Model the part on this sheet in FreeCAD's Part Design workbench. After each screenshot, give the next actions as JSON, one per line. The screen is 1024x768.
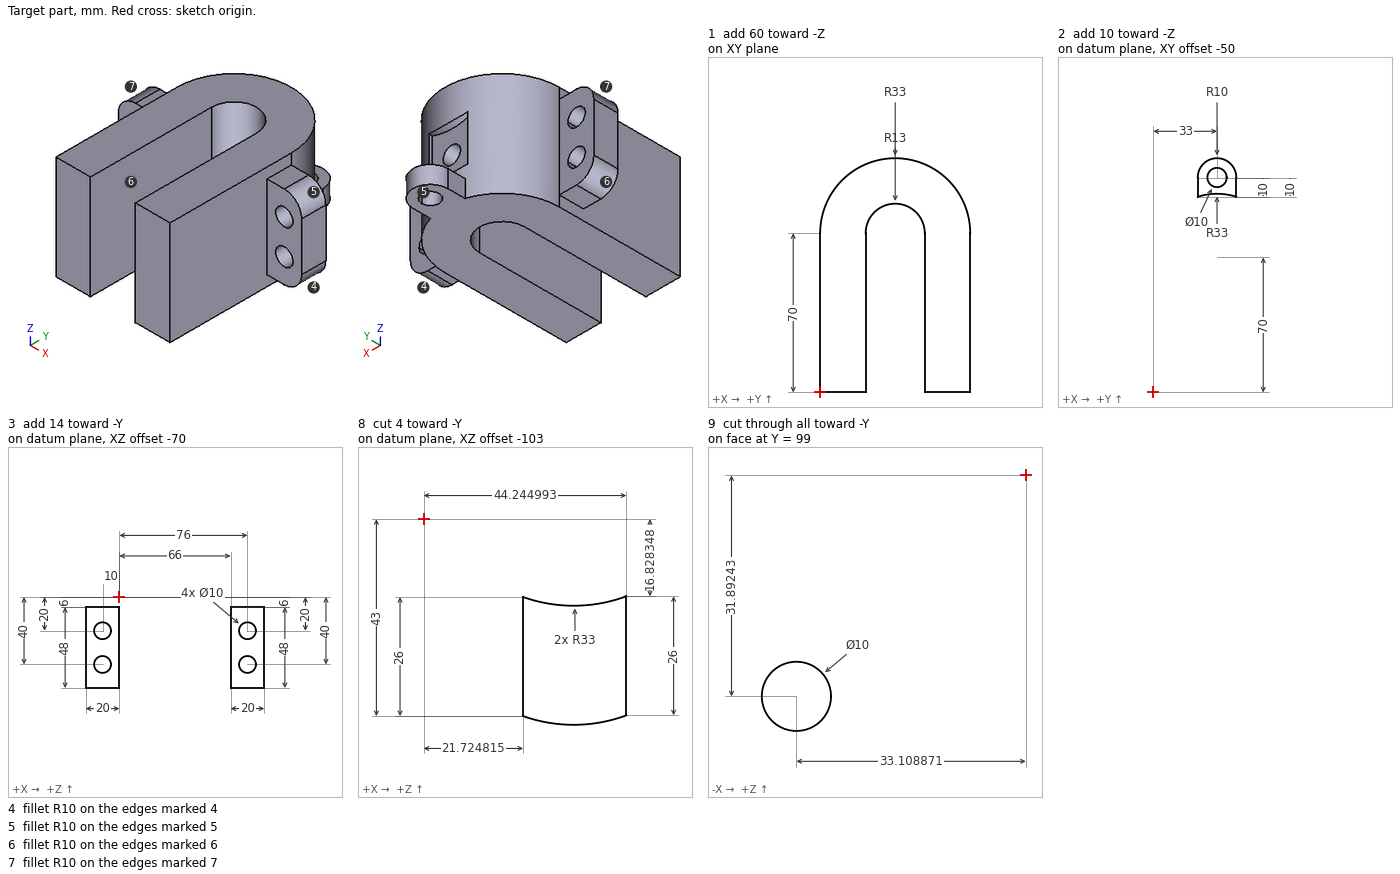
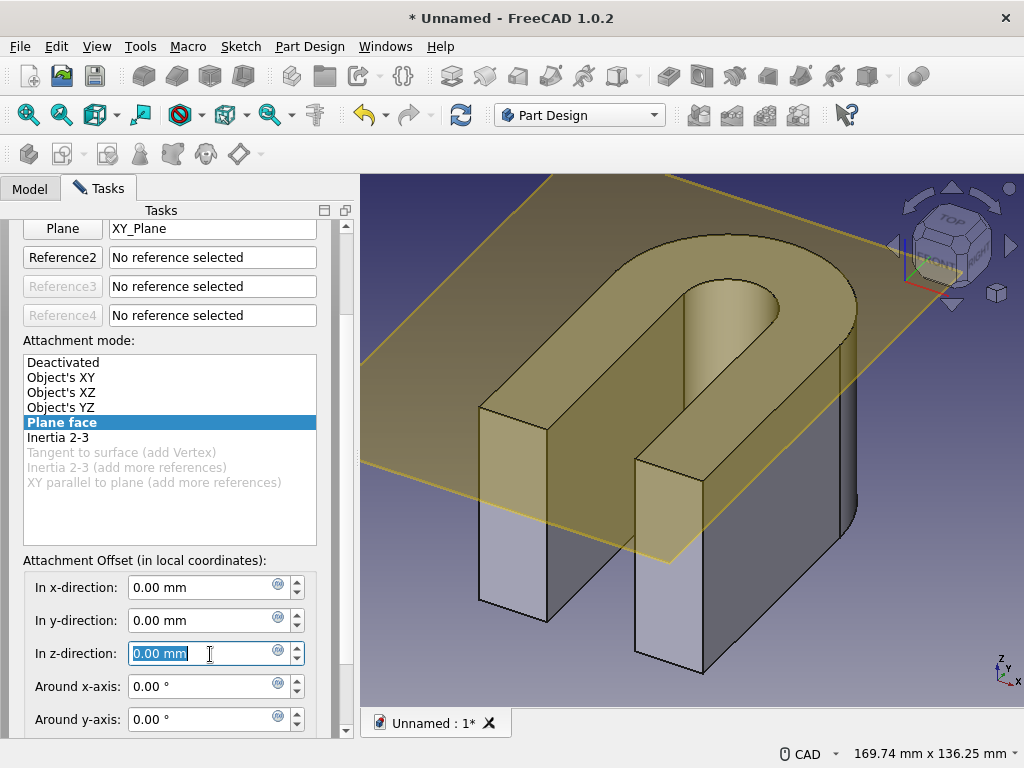
{"action": "type", "text": "-50"}
{"action": "key", "text": "Tab"}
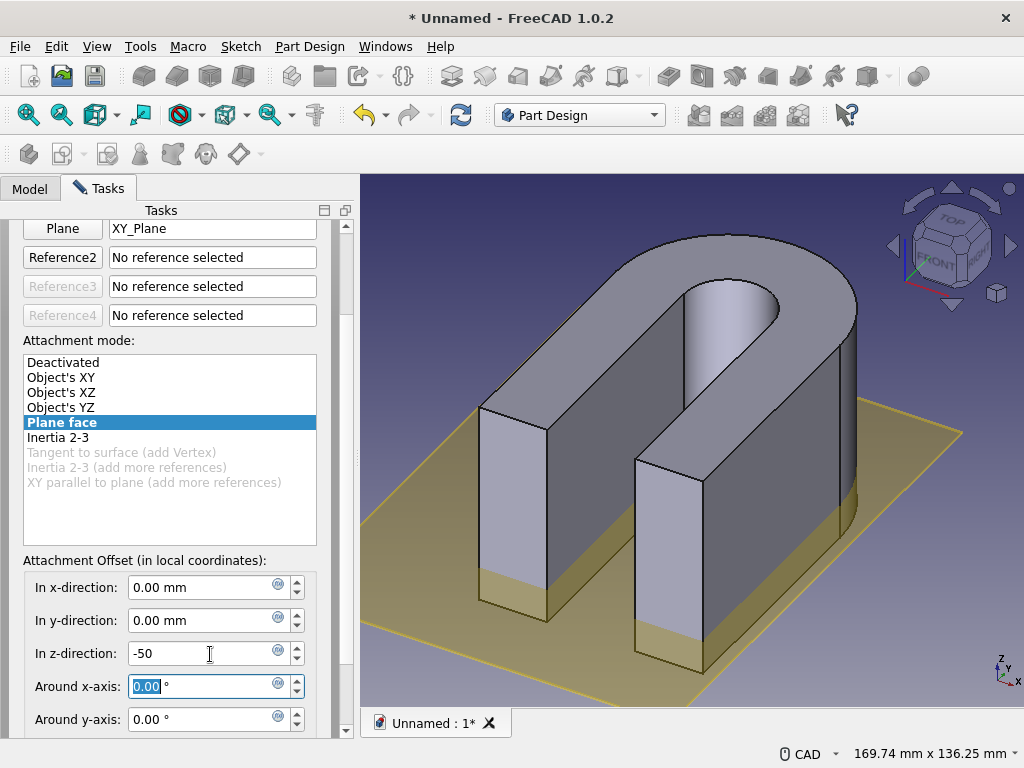
{"action": "scroll", "coordinate": [346, 479], "scroll_direction": "up", "scroll_amount": 3}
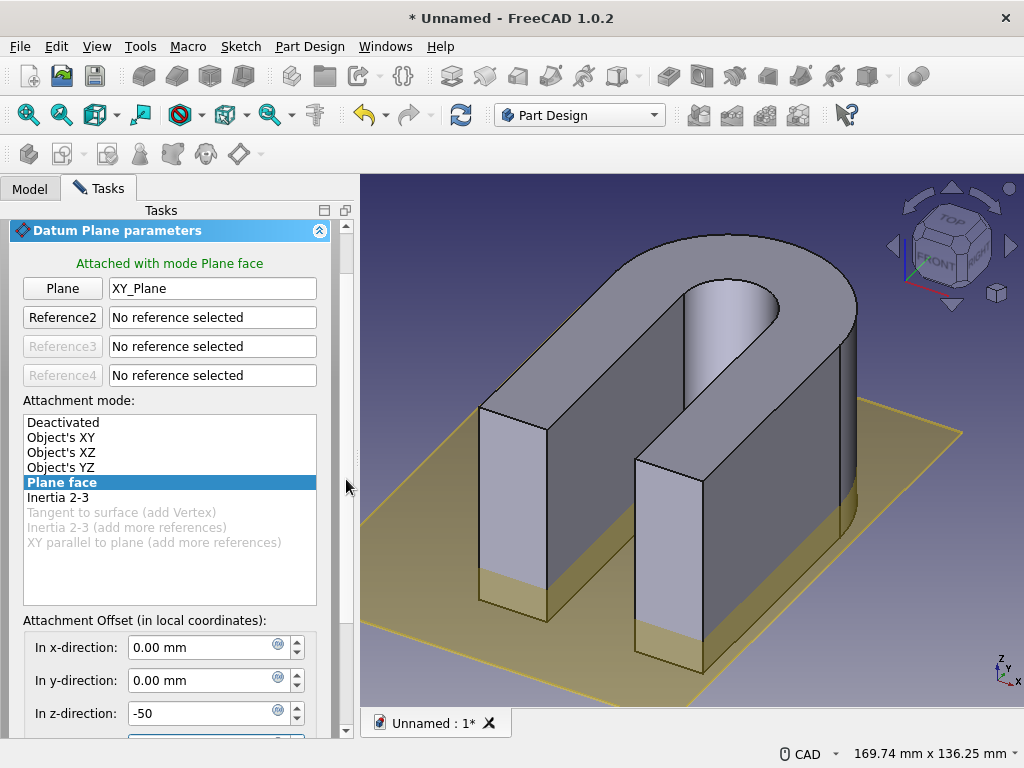
{"action": "left_click", "coordinate": [127, 249]}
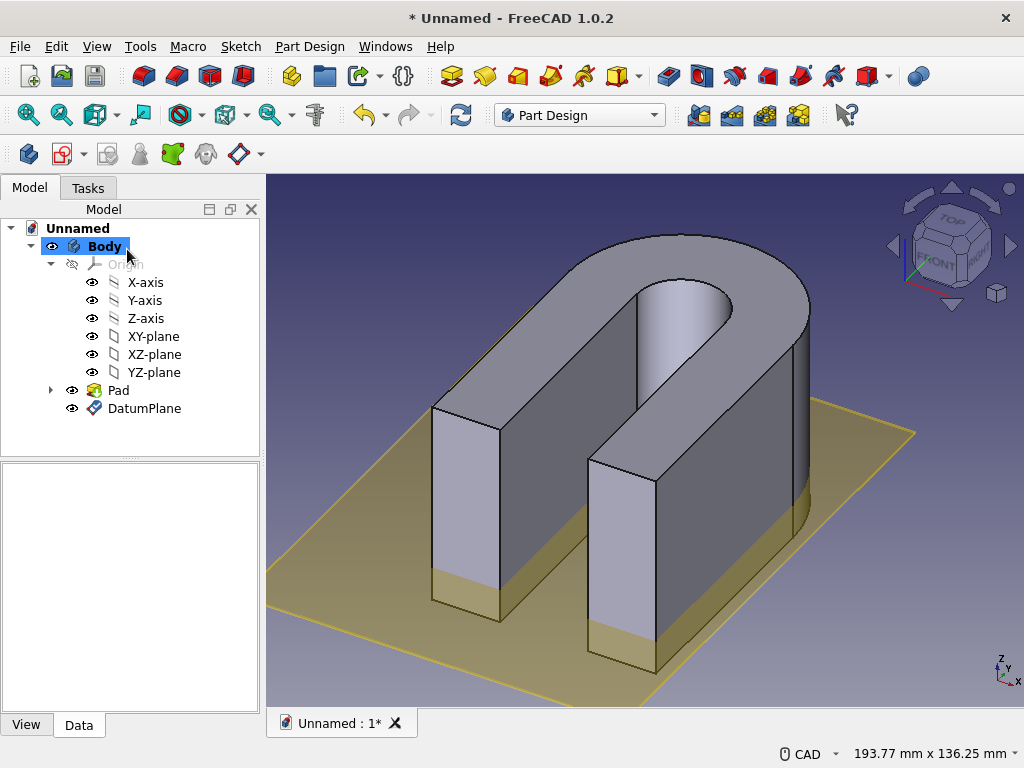
{"action": "left_click", "coordinate": [117, 408]}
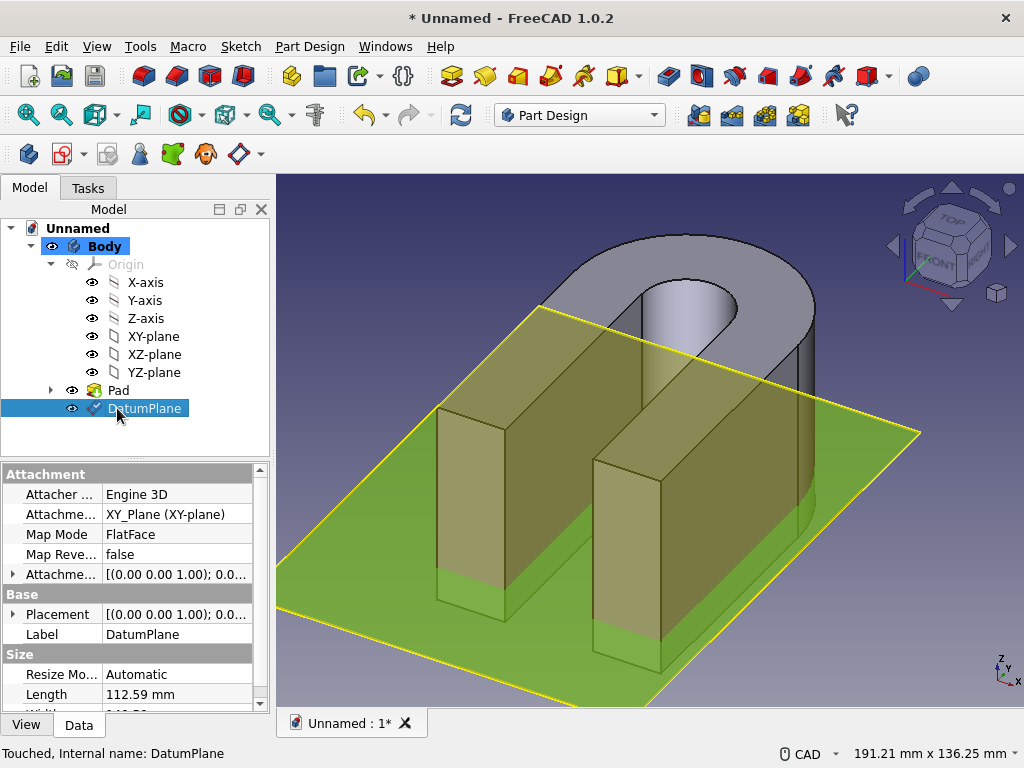
{"action": "left_click", "coordinate": [62, 154]}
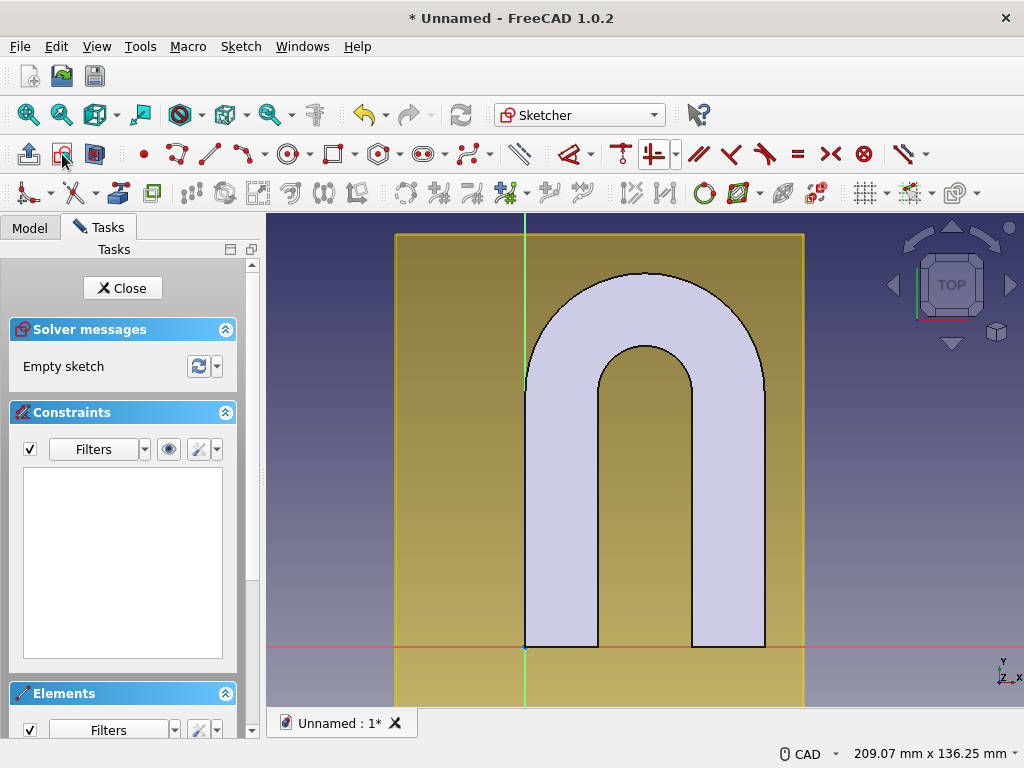
{"action": "key", "text": "q s"}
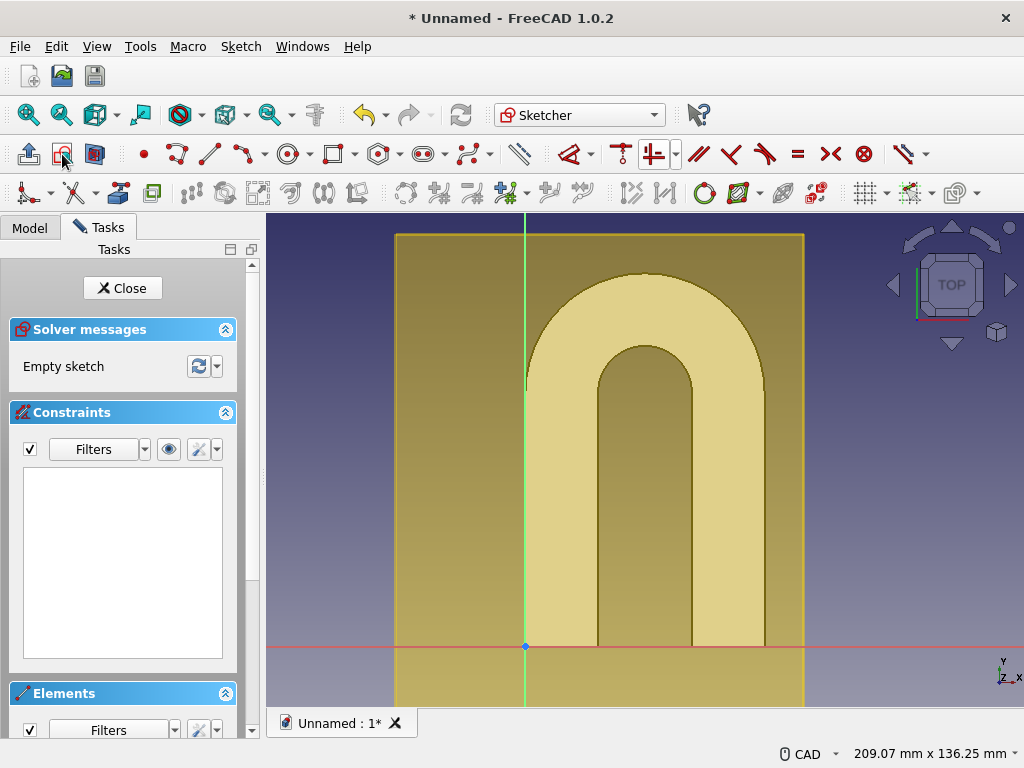
{"action": "scroll", "coordinate": [576, 460], "scroll_direction": "down", "scroll_amount": 5}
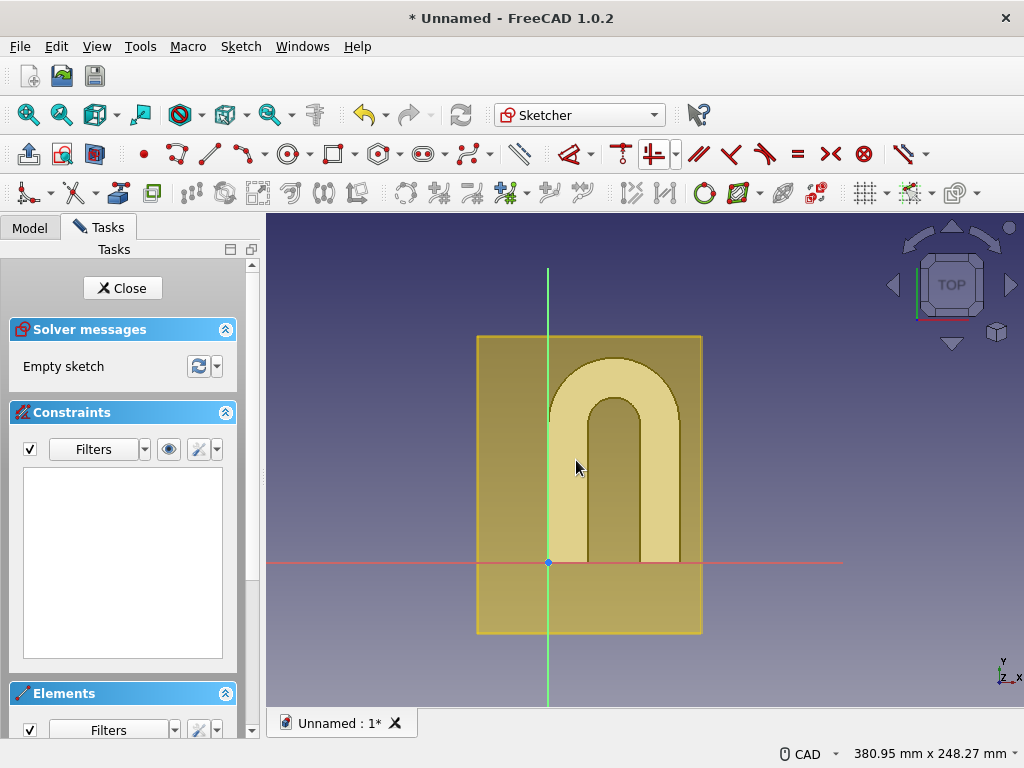
{"action": "scroll", "coordinate": [604, 372], "scroll_direction": "up", "scroll_amount": 12}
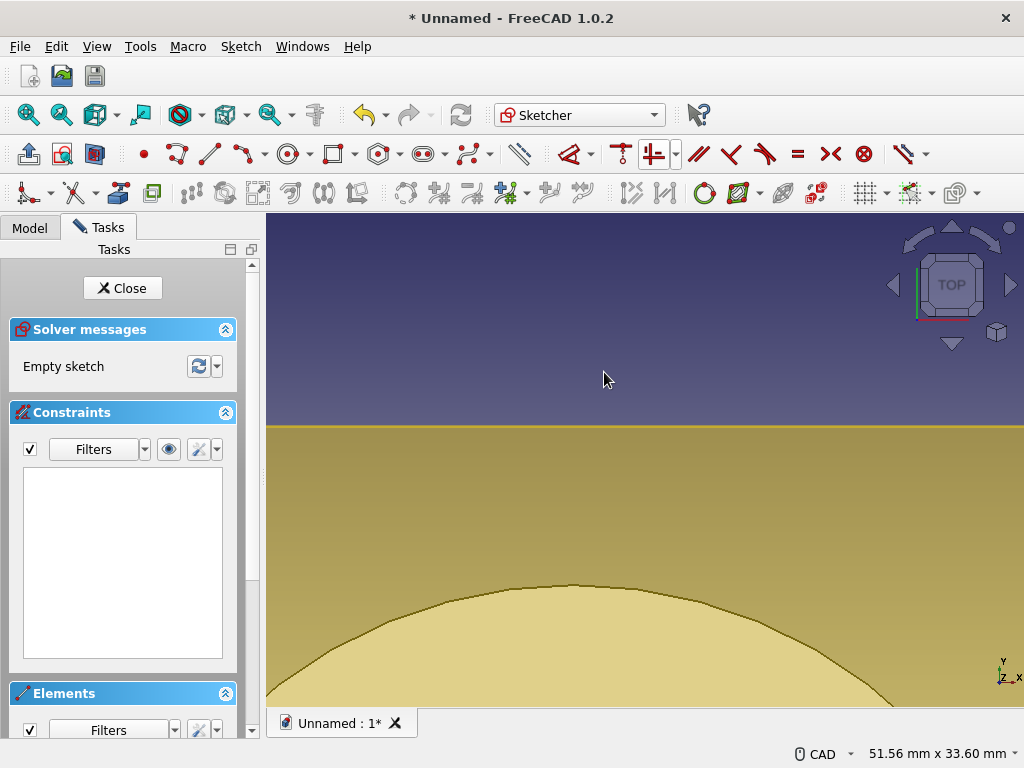
{"action": "key", "text": "g l"}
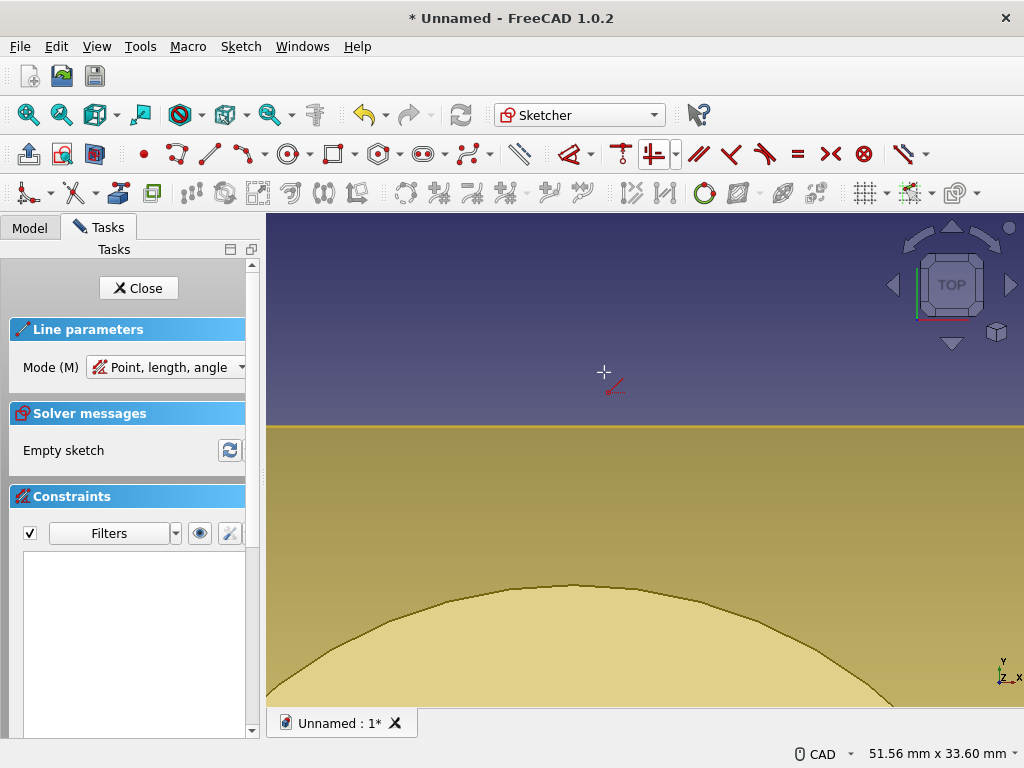
{"action": "left_click", "coordinate": [721, 461]}
{"action": "left_click", "coordinate": [721, 608]}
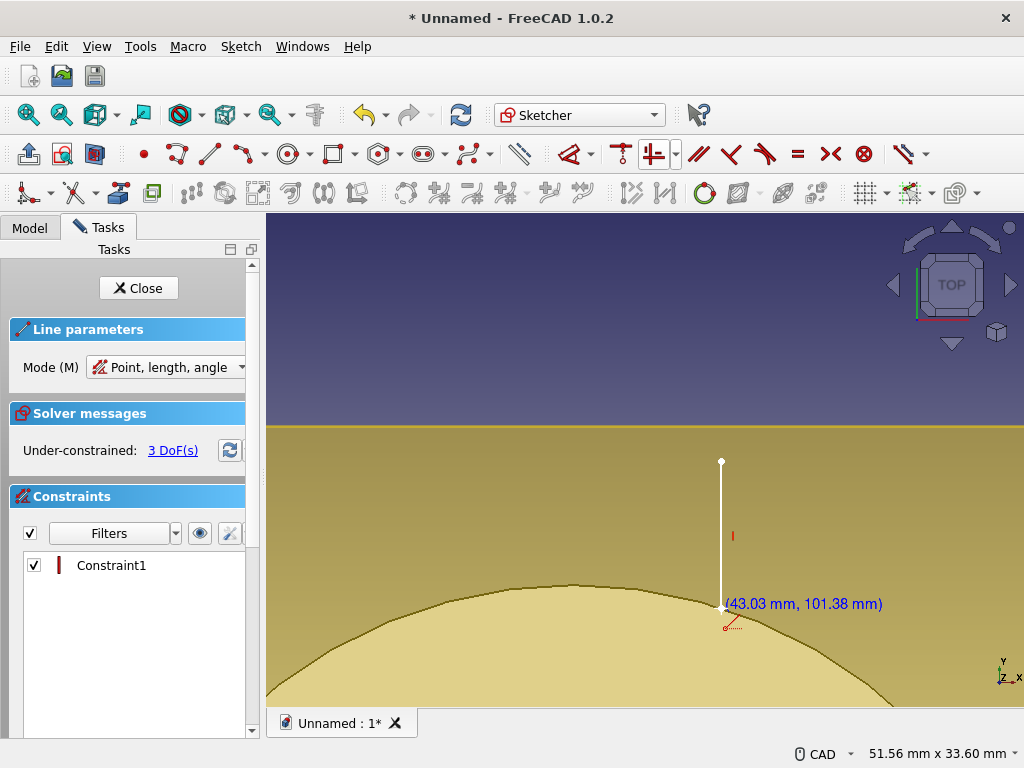
{"action": "left_click", "coordinate": [427, 608]}
{"action": "left_click", "coordinate": [427, 461]}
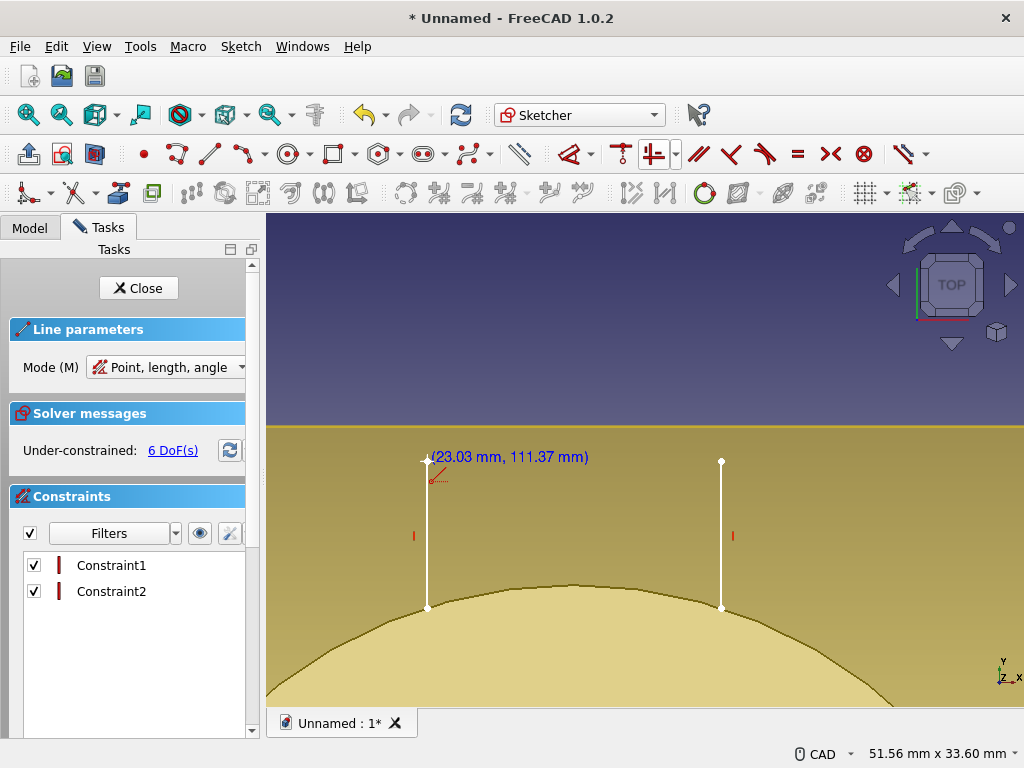
{"action": "left_click", "coordinate": [242, 154]}